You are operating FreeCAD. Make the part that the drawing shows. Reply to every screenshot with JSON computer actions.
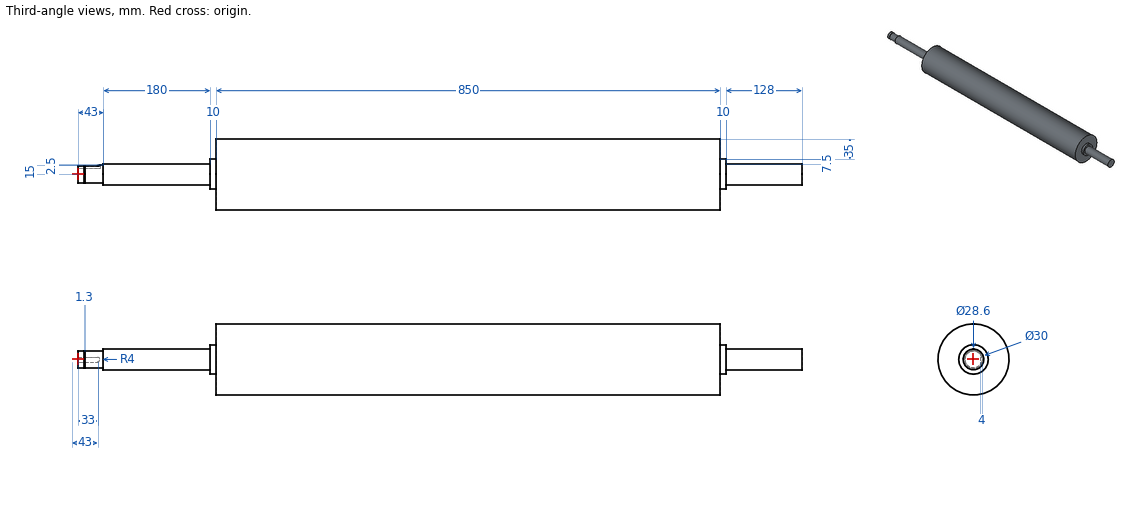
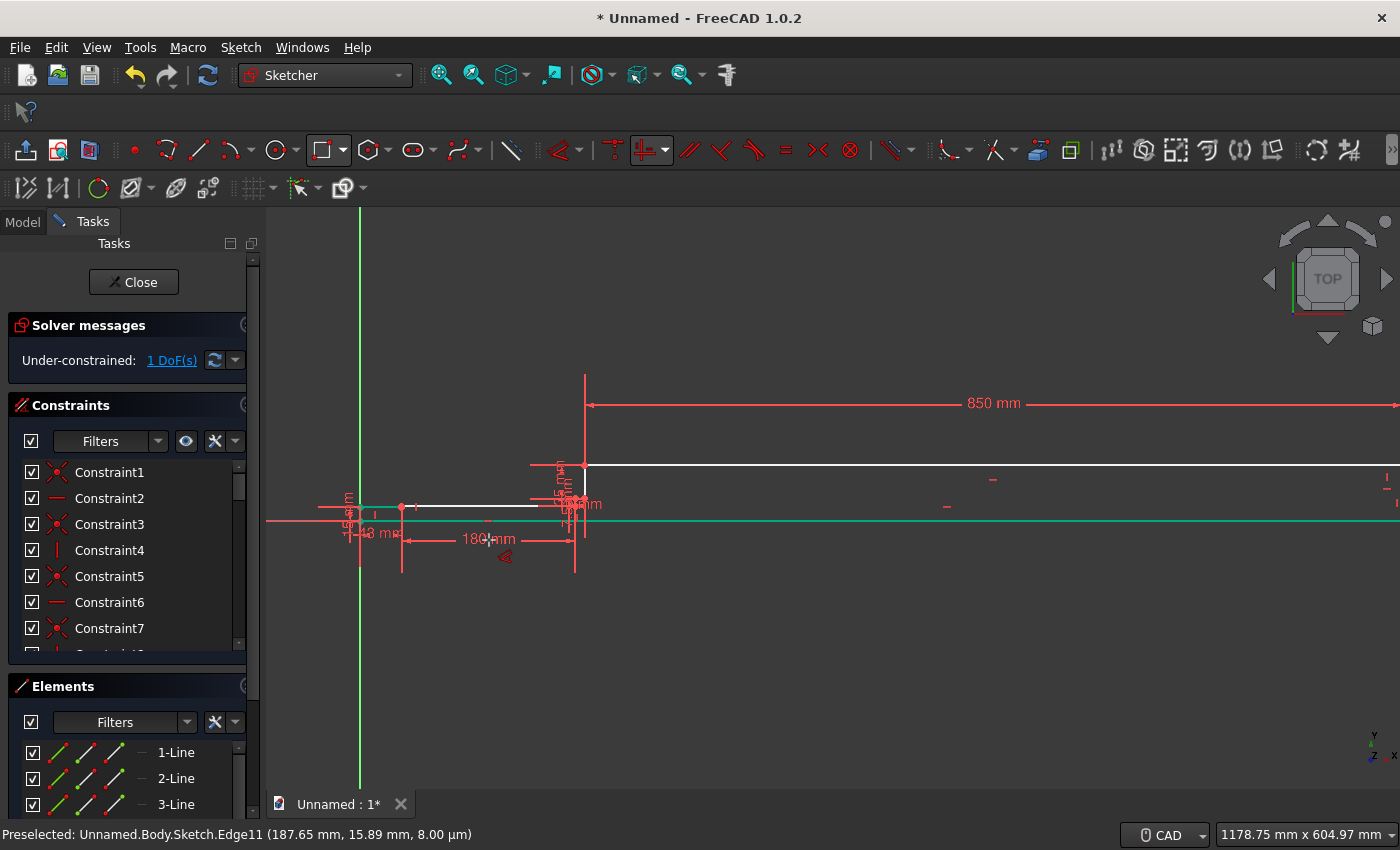
{"action": "scroll", "coordinate": [402, 507], "scroll_direction": "up", "scroll_amount": 15}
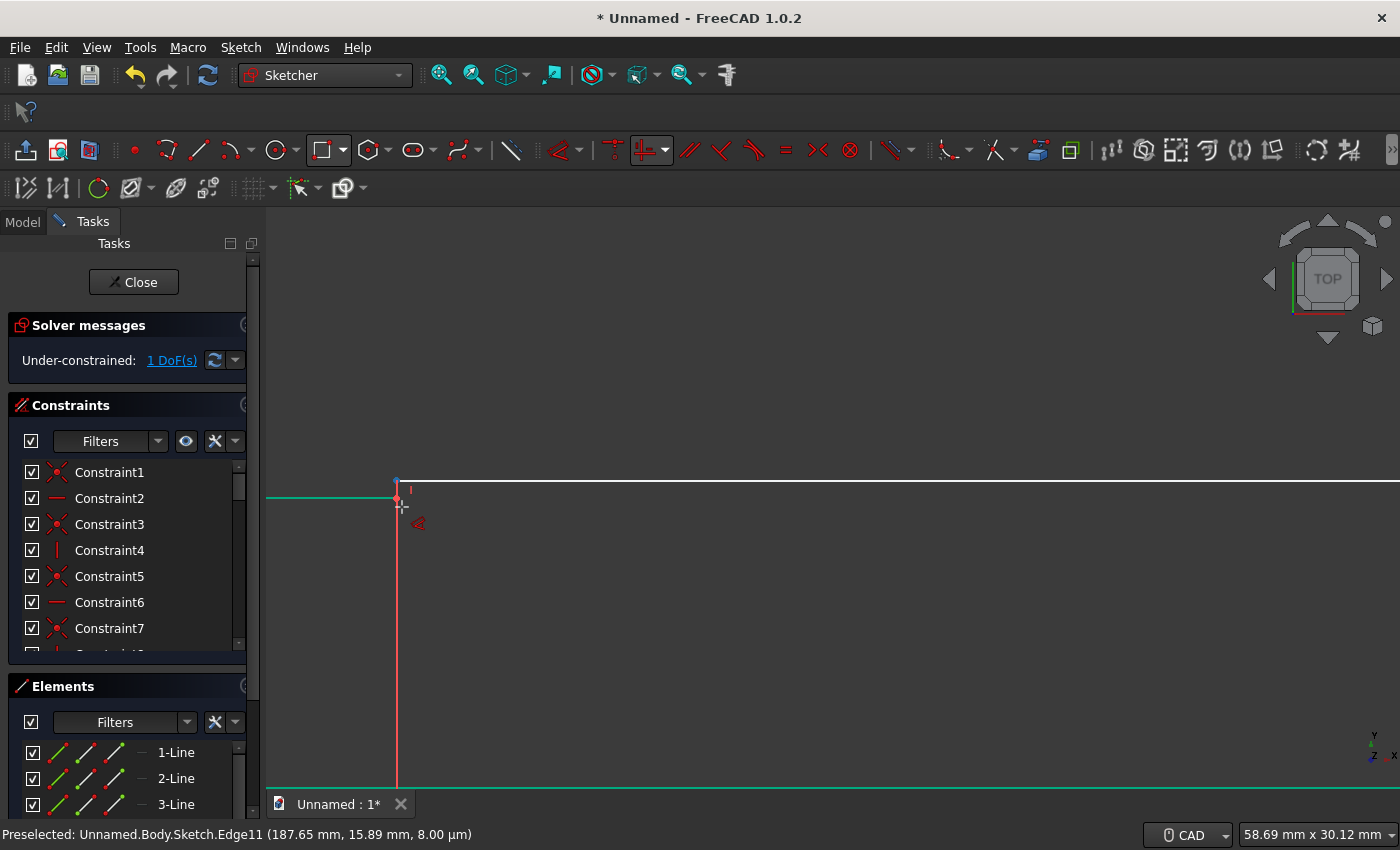
{"action": "left_click", "coordinate": [397, 489]}
{"action": "left_click", "coordinate": [363, 483]}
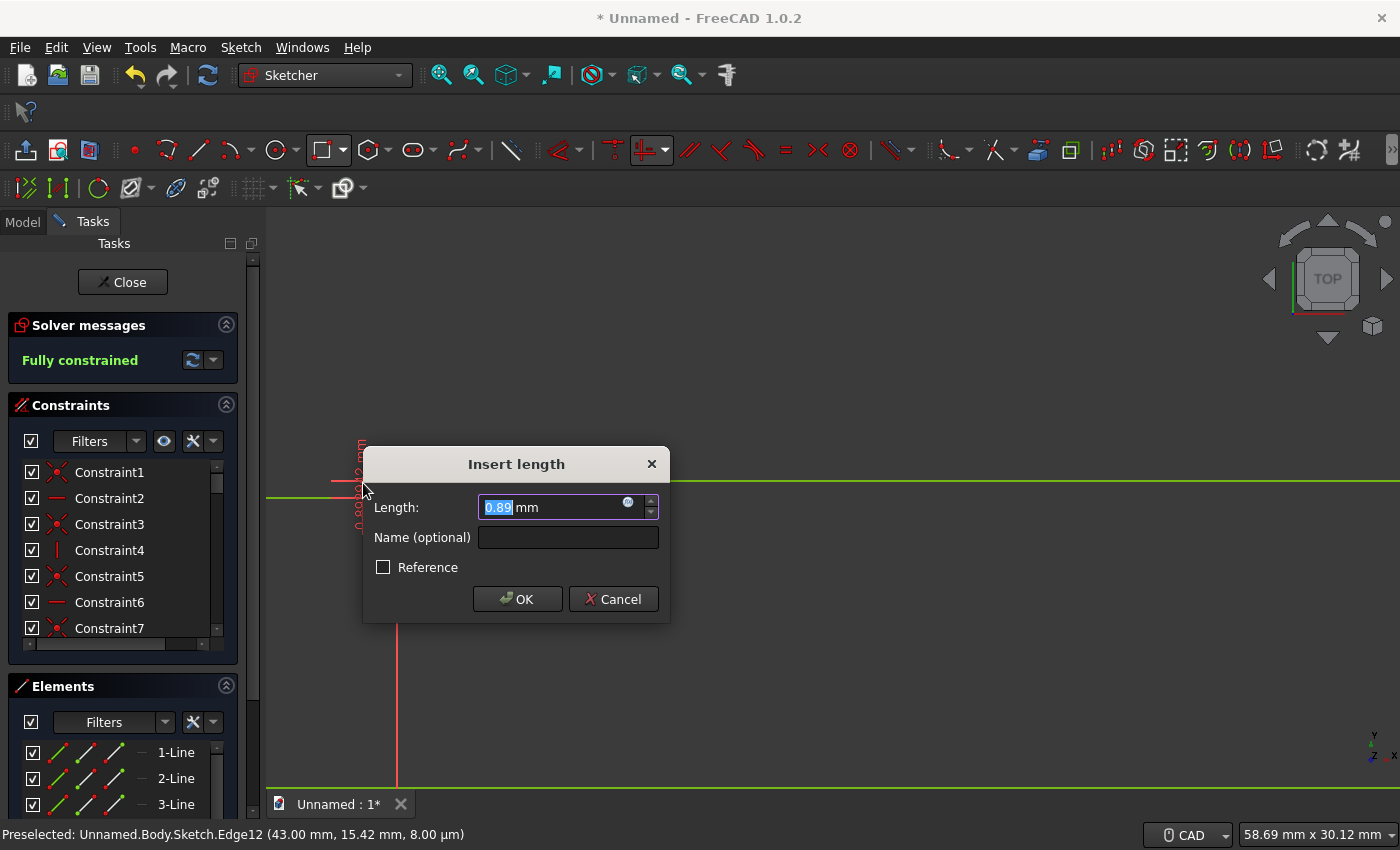
{"action": "type", "text": "2.5"}
{"action": "key", "text": "Return"}
{"action": "key", "text": "Escape"}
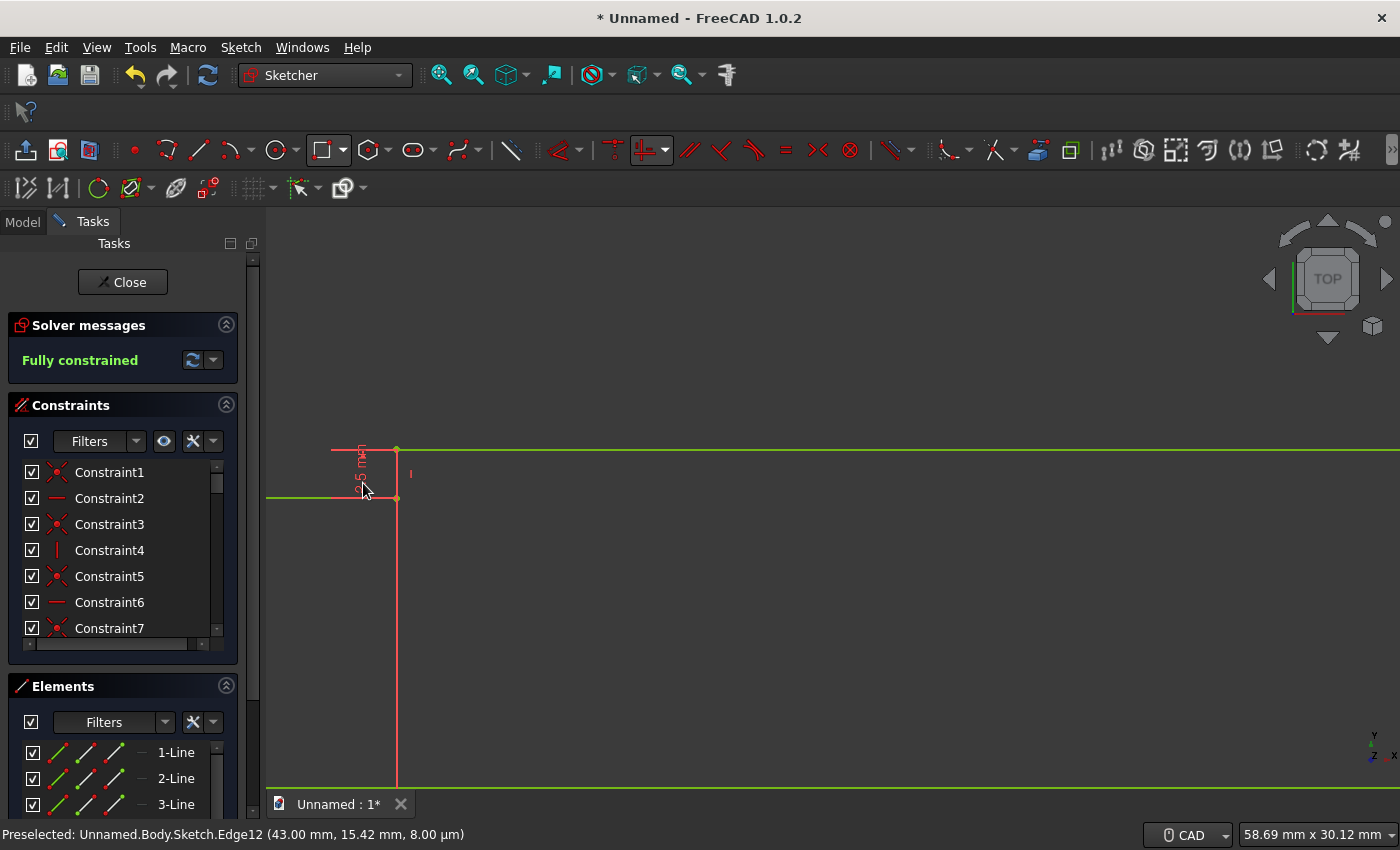
{"action": "left_click", "coordinate": [123, 282]}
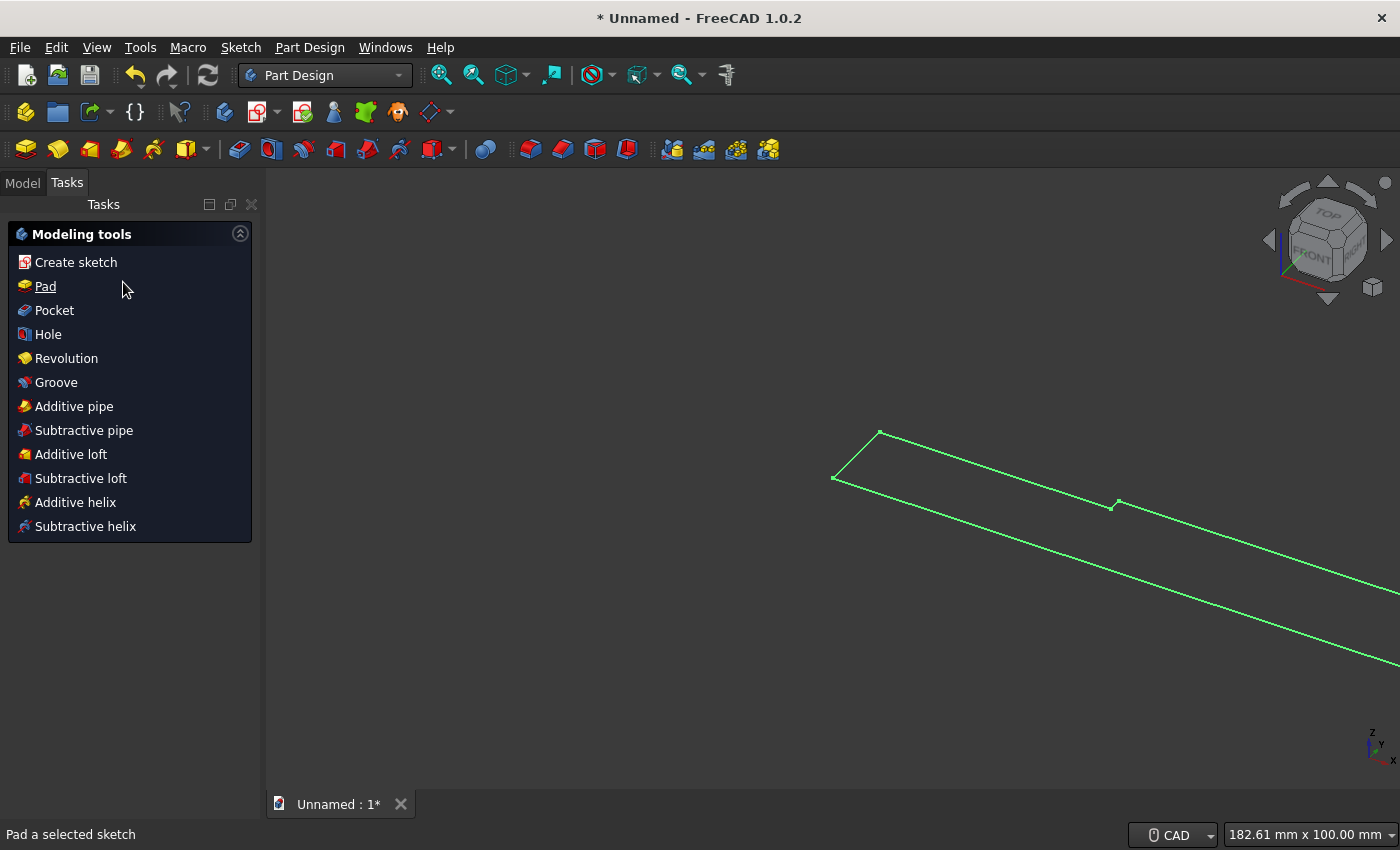
{"action": "left_click", "coordinate": [58, 150]}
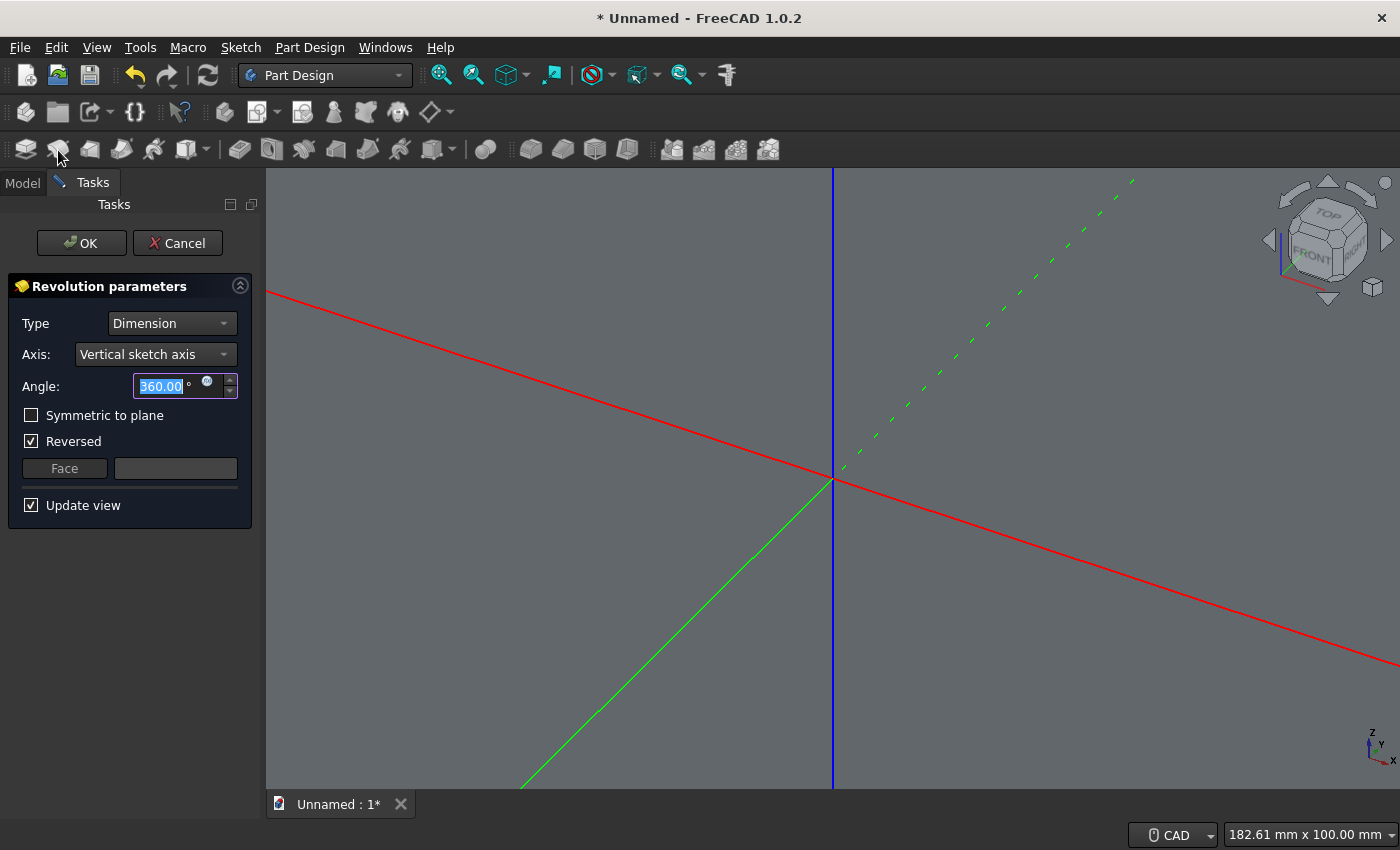
{"action": "left_click", "coordinate": [156, 354]}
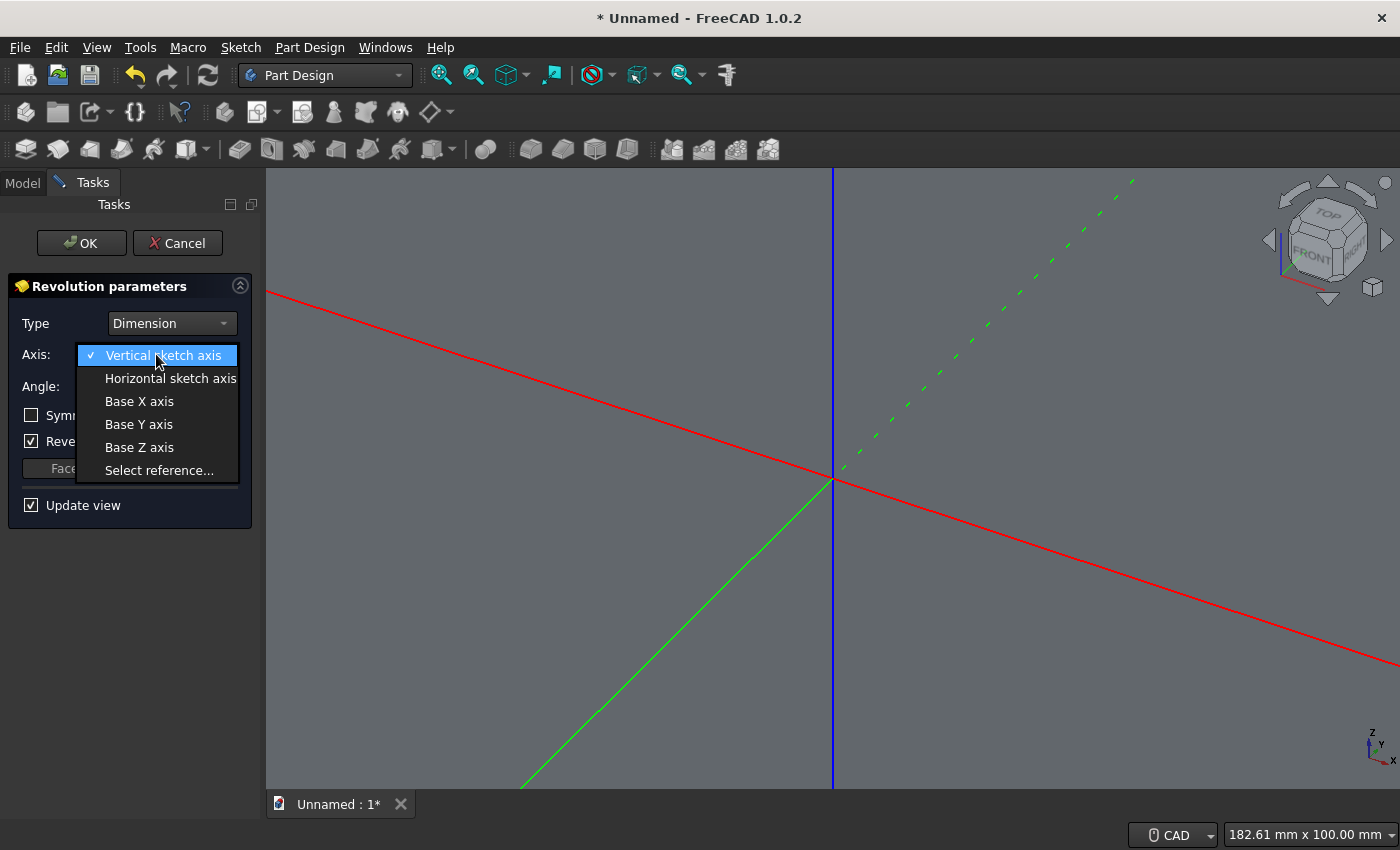
{"action": "left_click", "coordinate": [156, 378]}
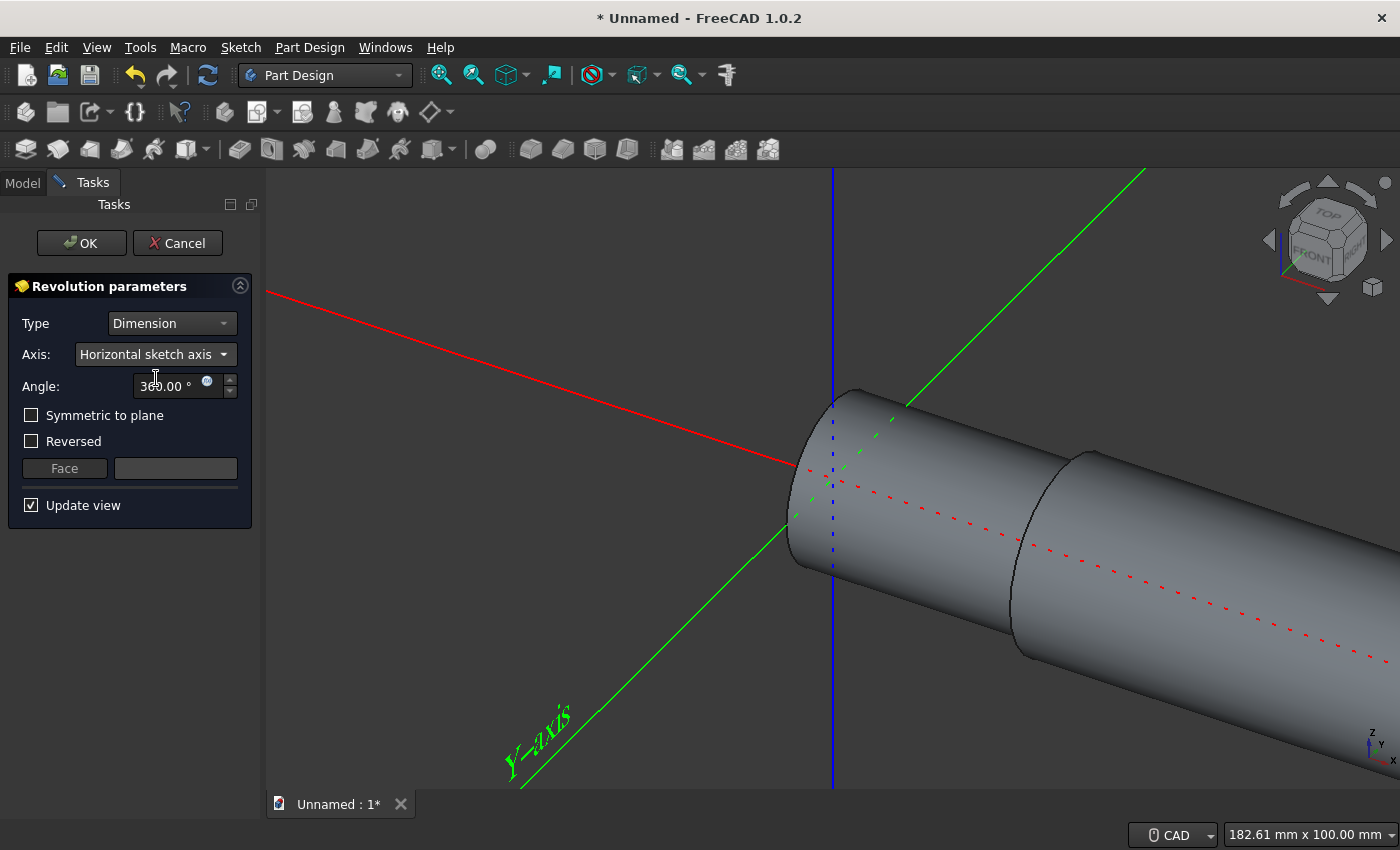
{"action": "left_click", "coordinate": [82, 243]}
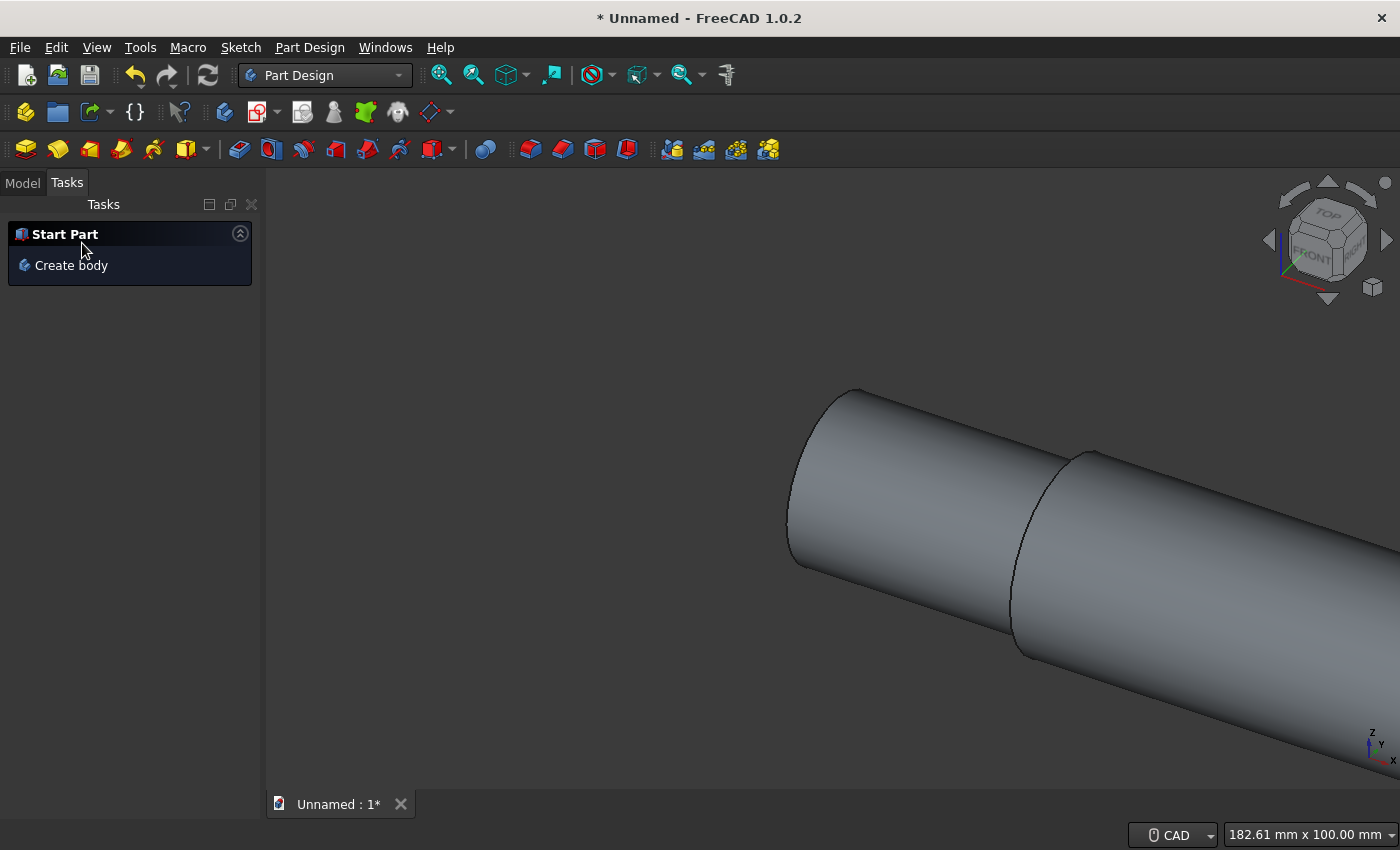
{"action": "left_click", "coordinate": [442, 76]}